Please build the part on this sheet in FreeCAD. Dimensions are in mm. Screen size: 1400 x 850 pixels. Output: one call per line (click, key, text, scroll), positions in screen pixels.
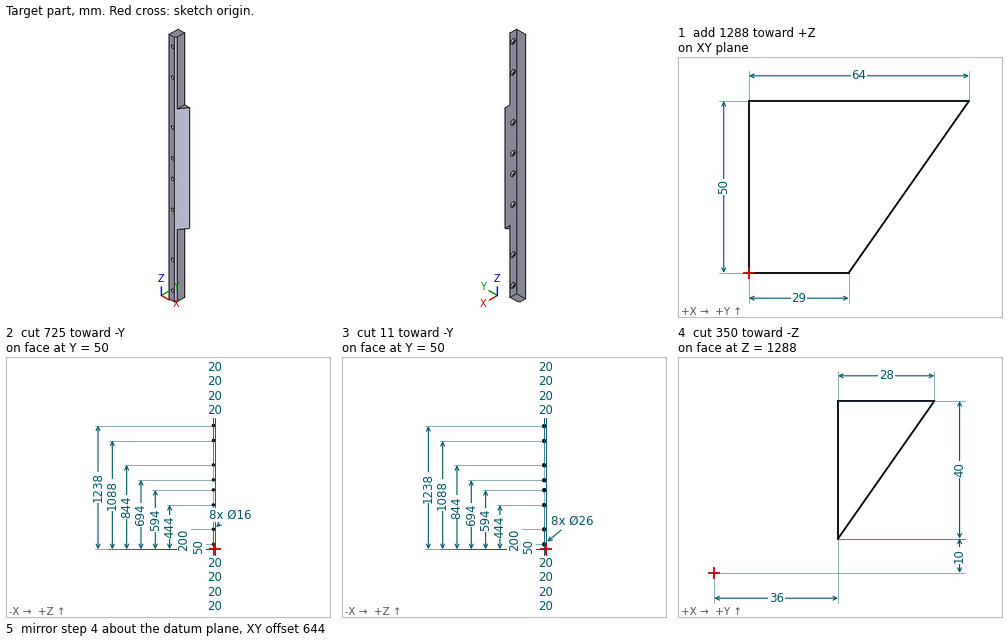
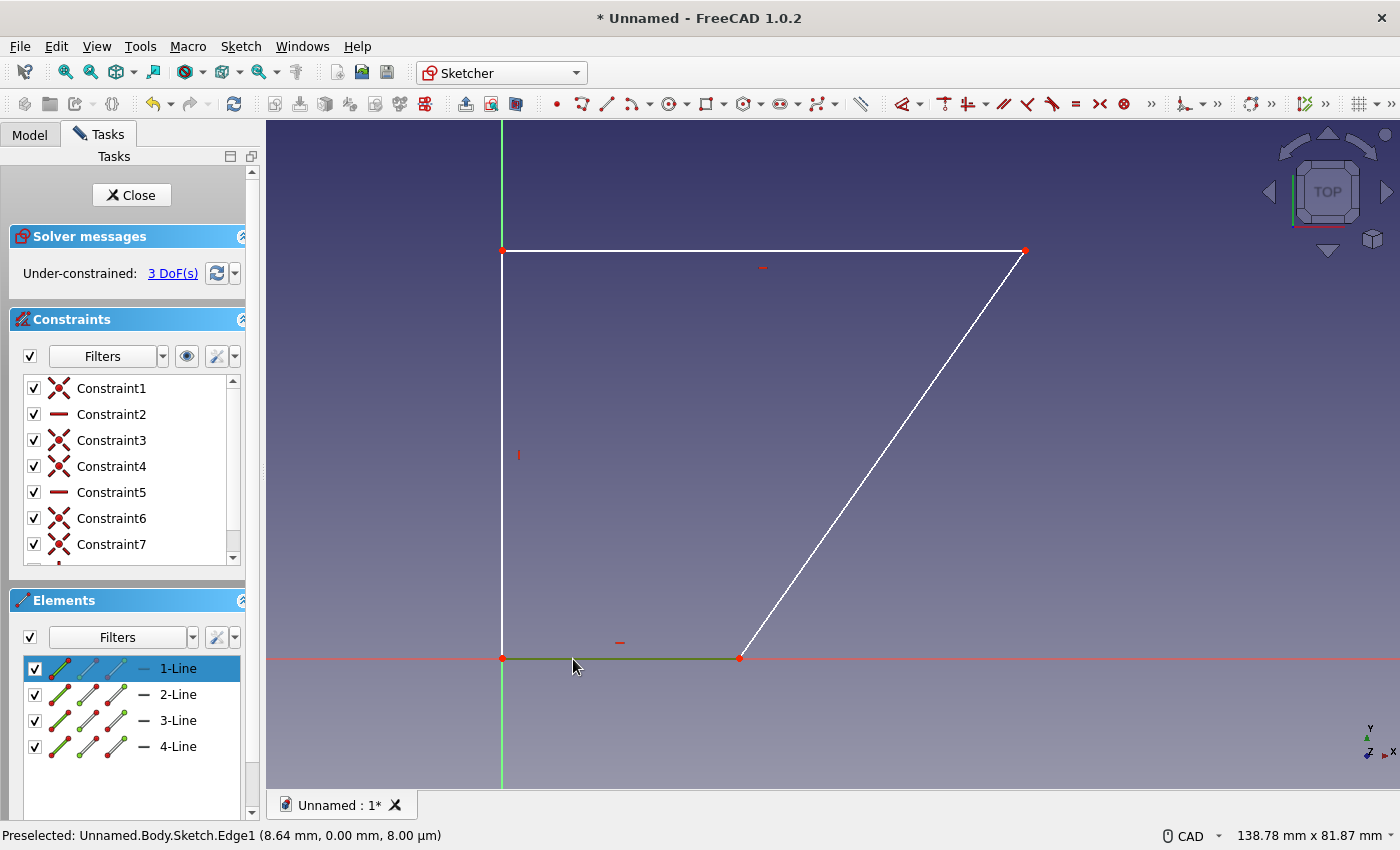
key(l)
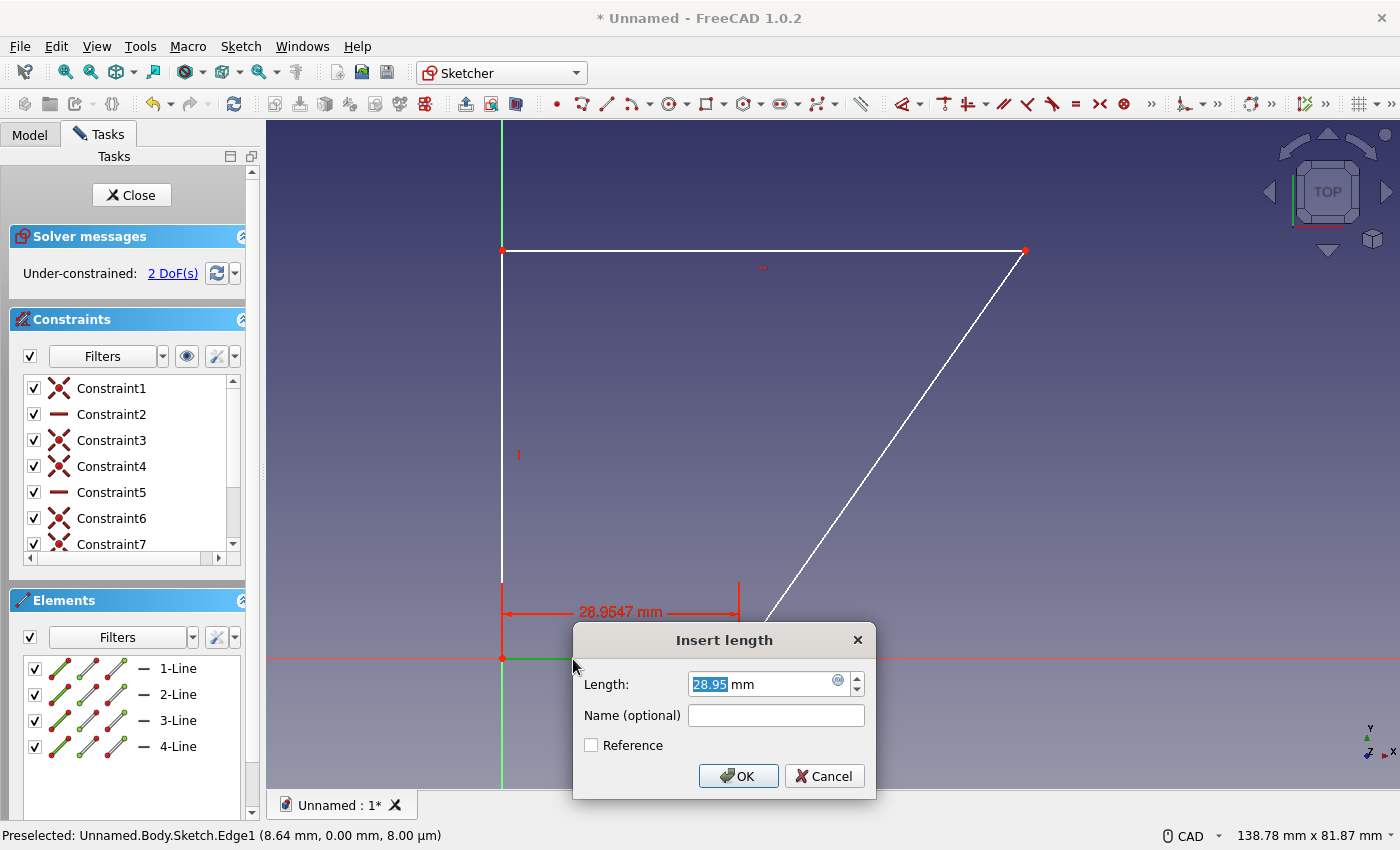
text(29)
key(Return)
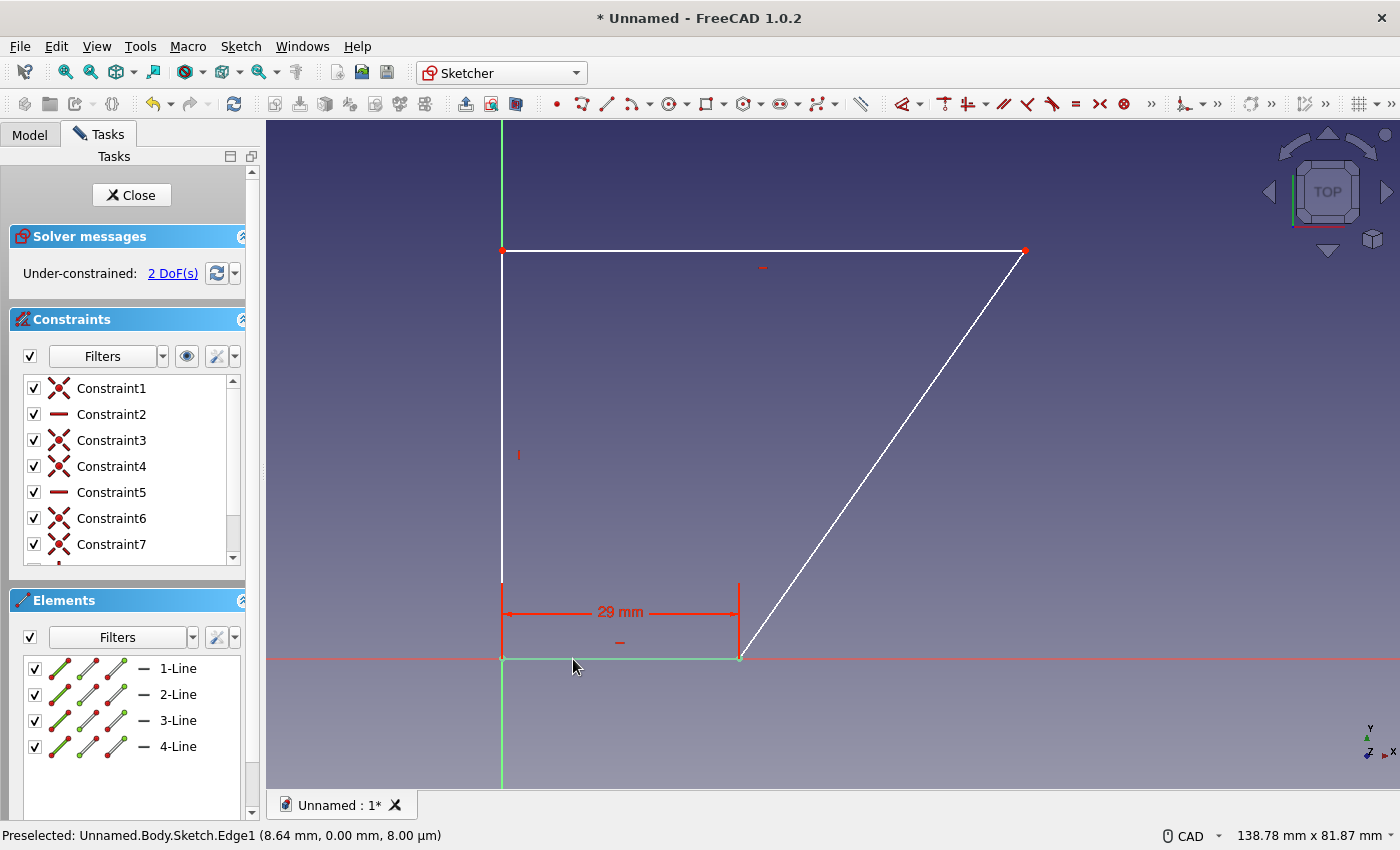
click(868, 251)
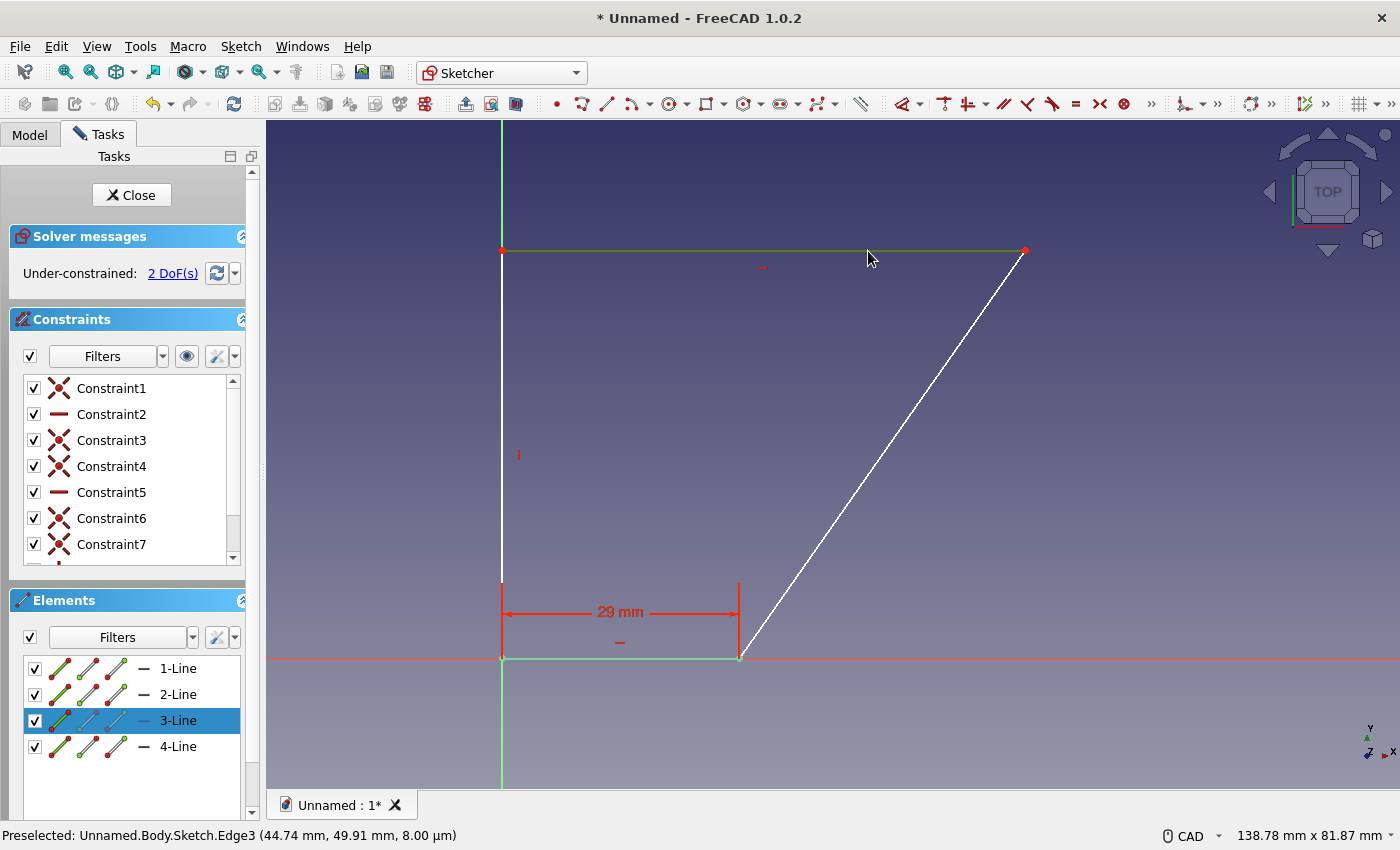
key(l)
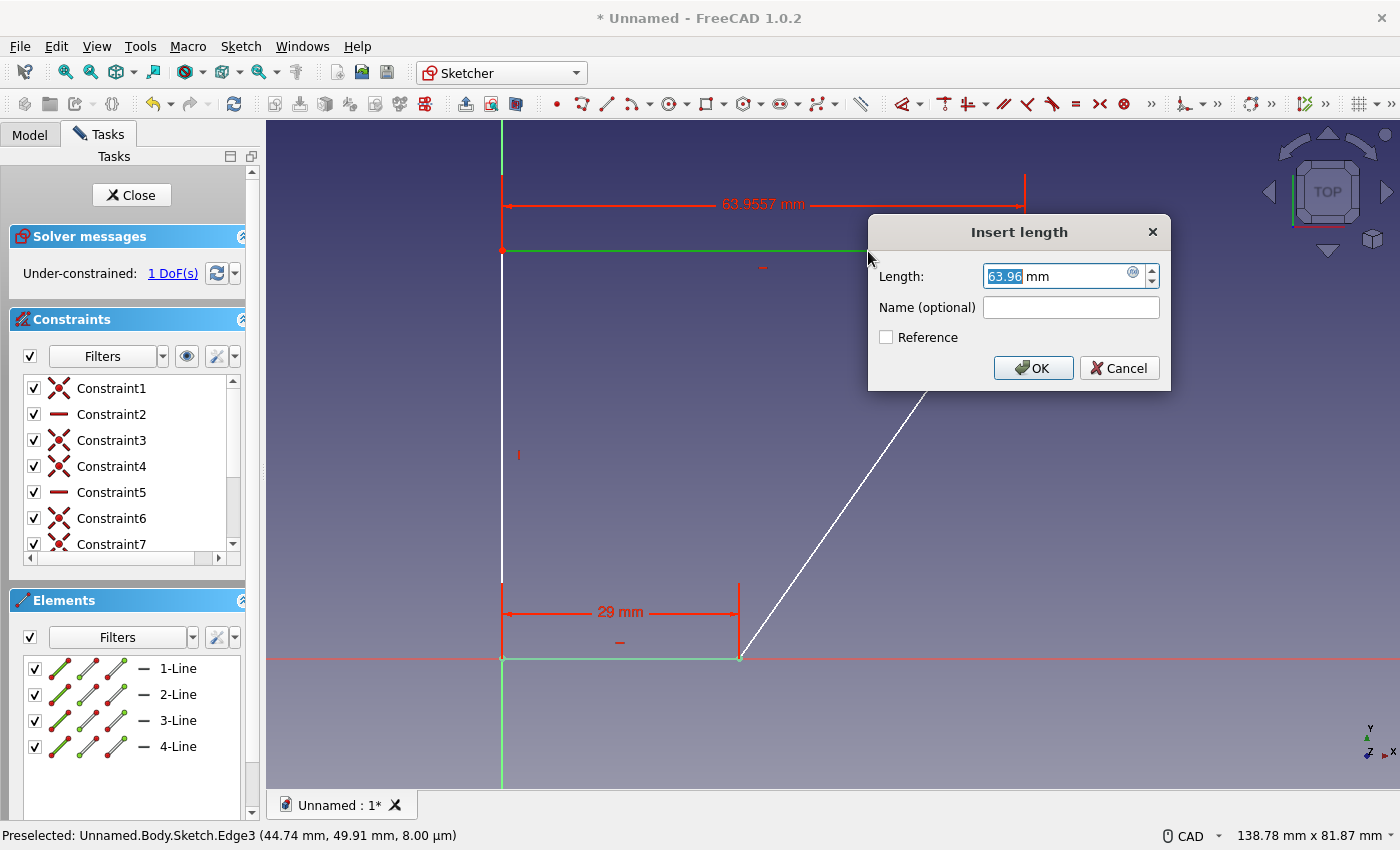
text(64)
key(Return)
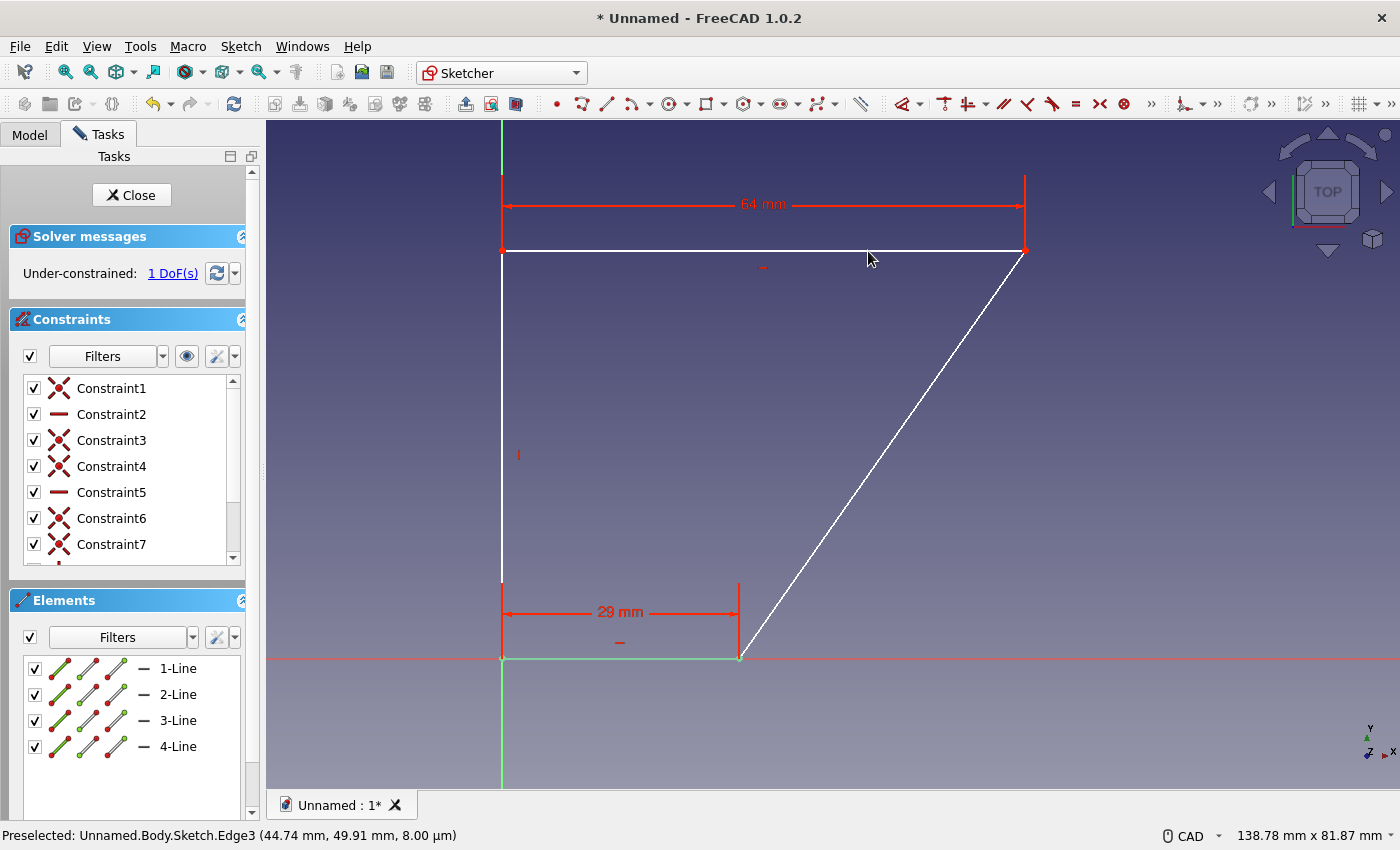
click(502, 373)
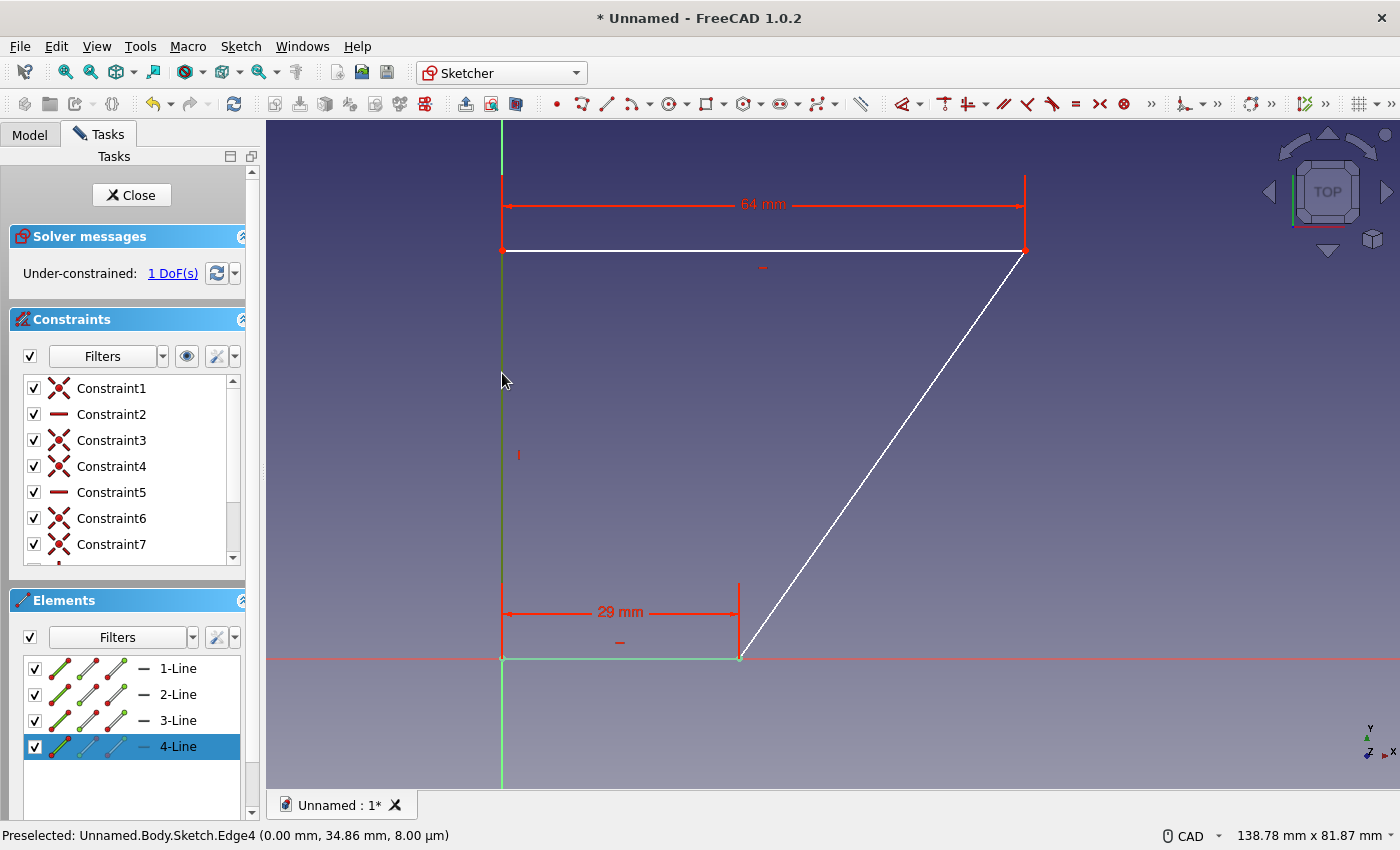
key(i)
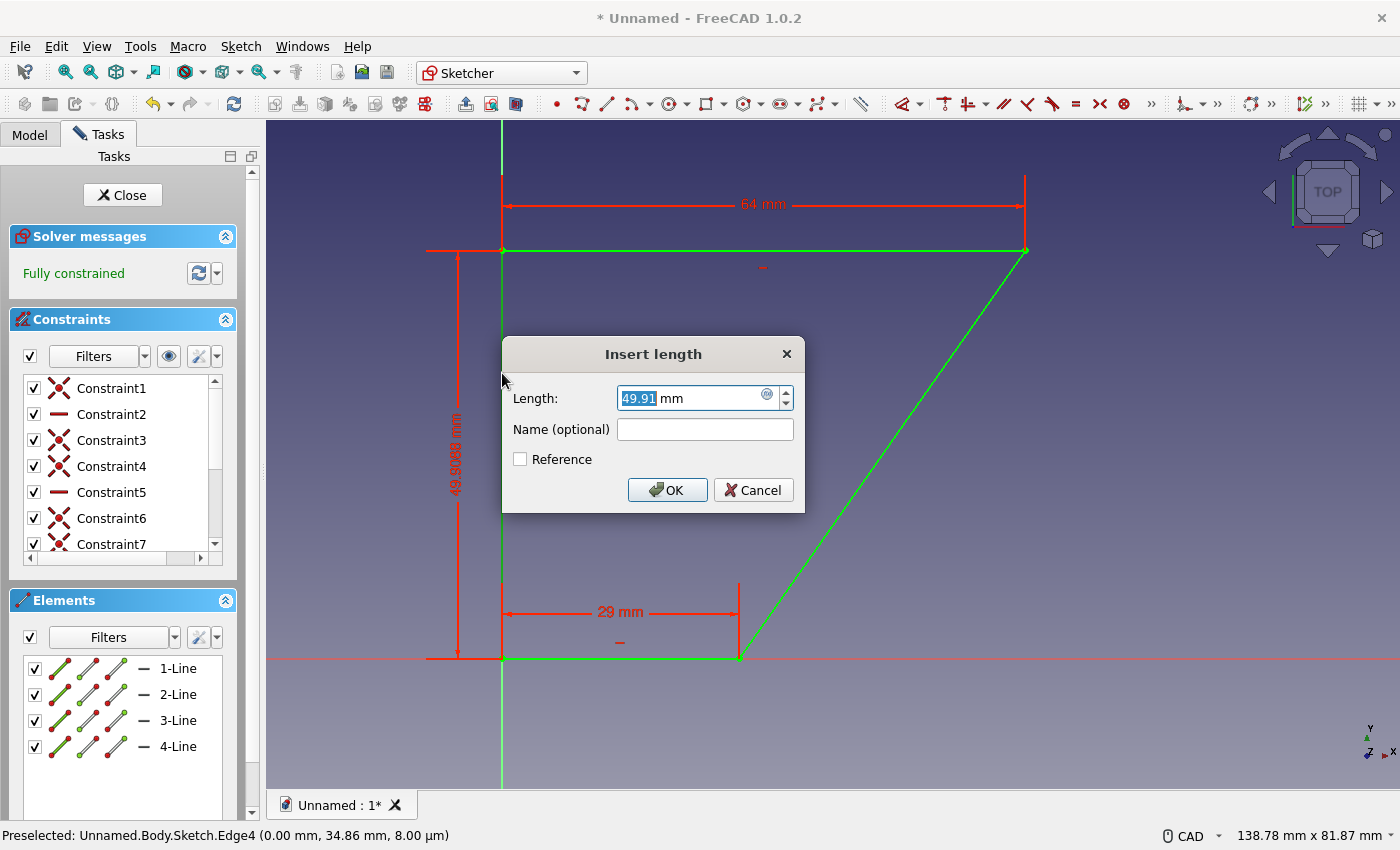
text(50)
key(Return)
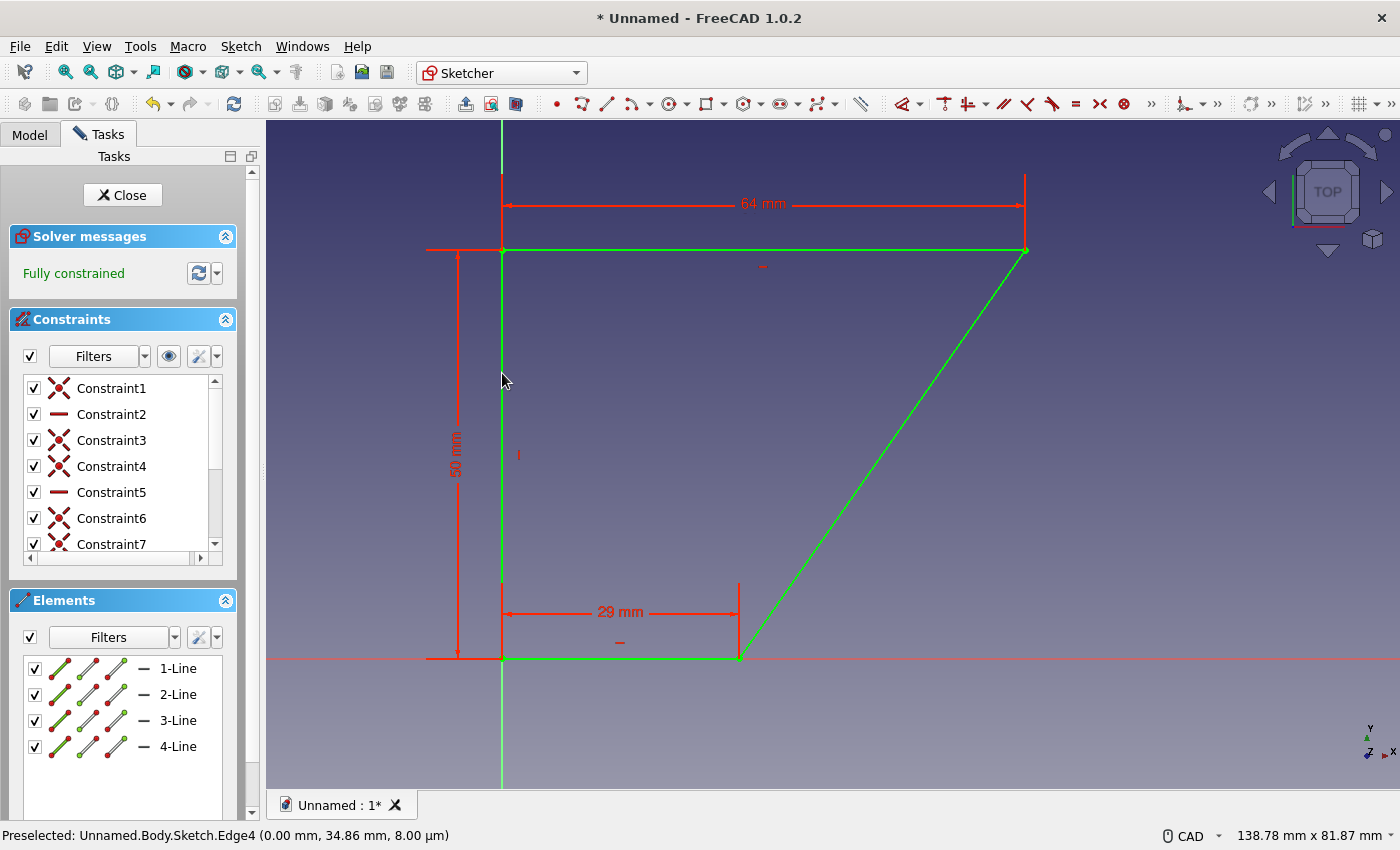
click(123, 195)